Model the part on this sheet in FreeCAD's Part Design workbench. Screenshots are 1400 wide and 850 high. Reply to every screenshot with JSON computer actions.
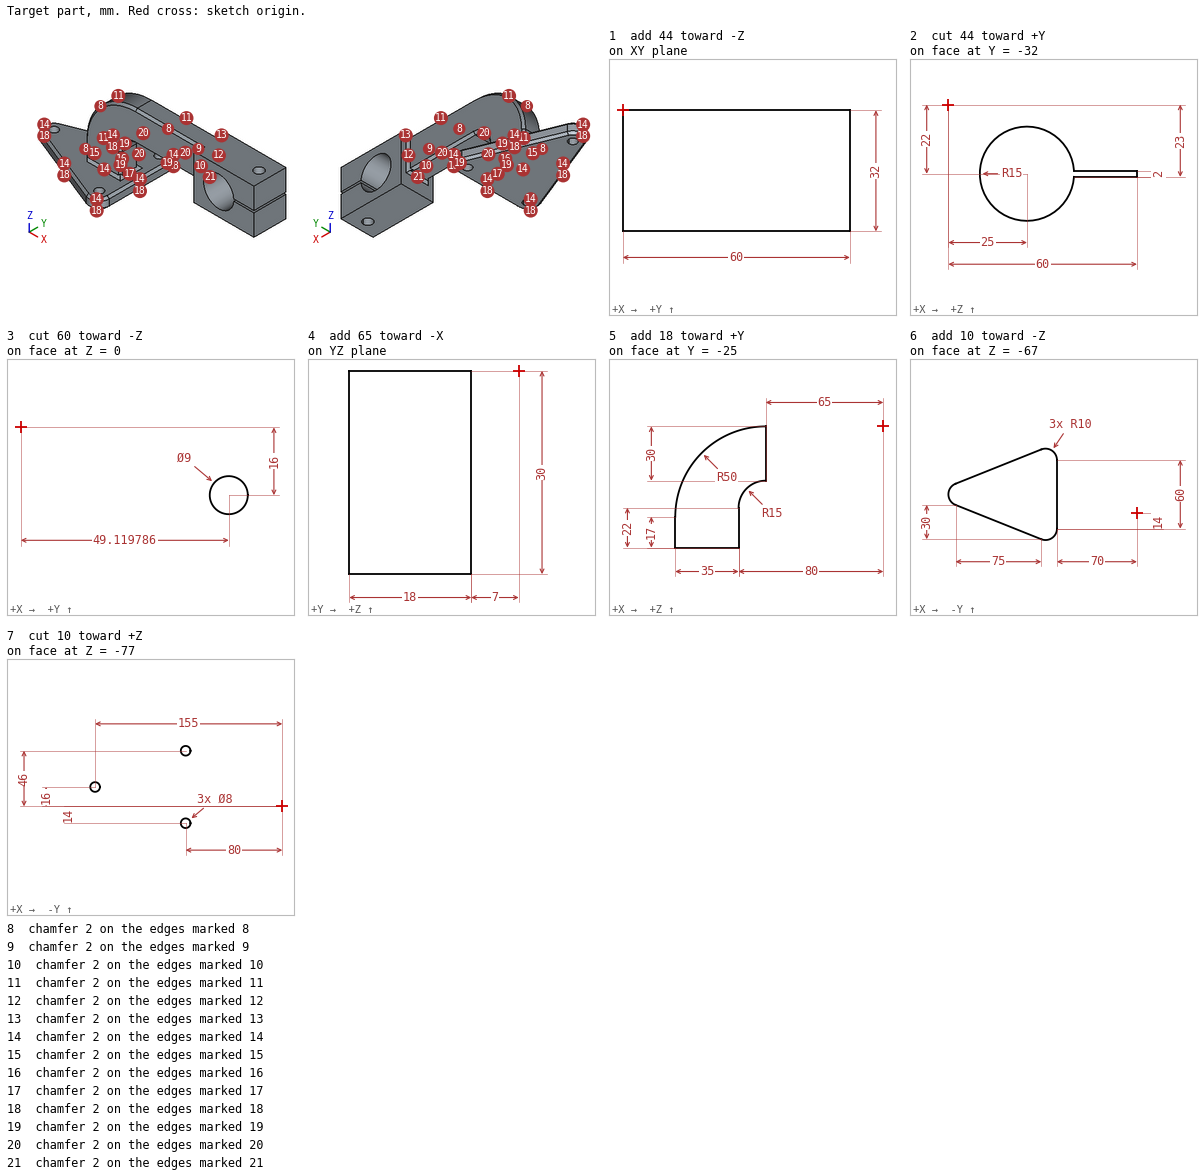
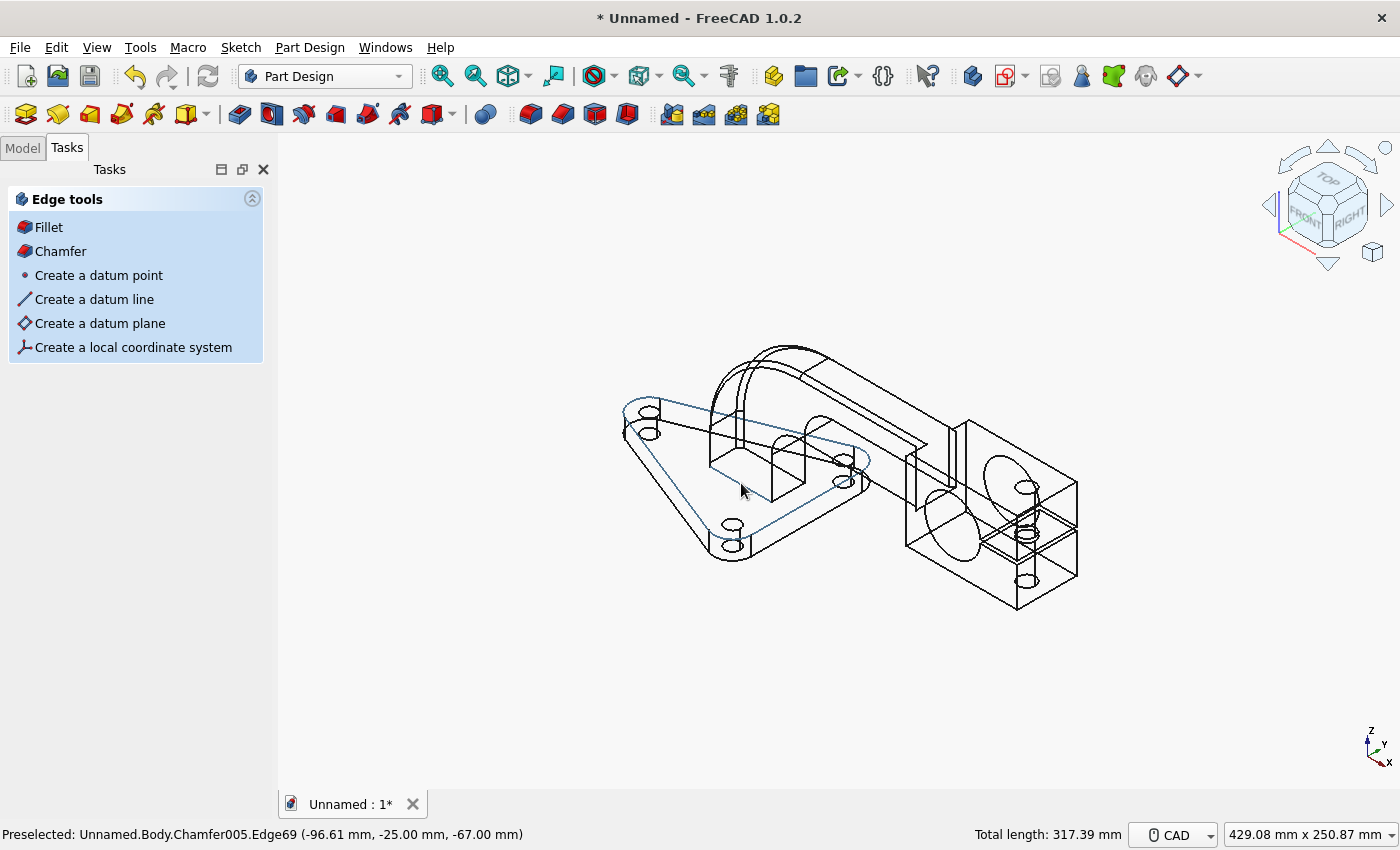
{"action": "left_click", "coordinate": [564, 114]}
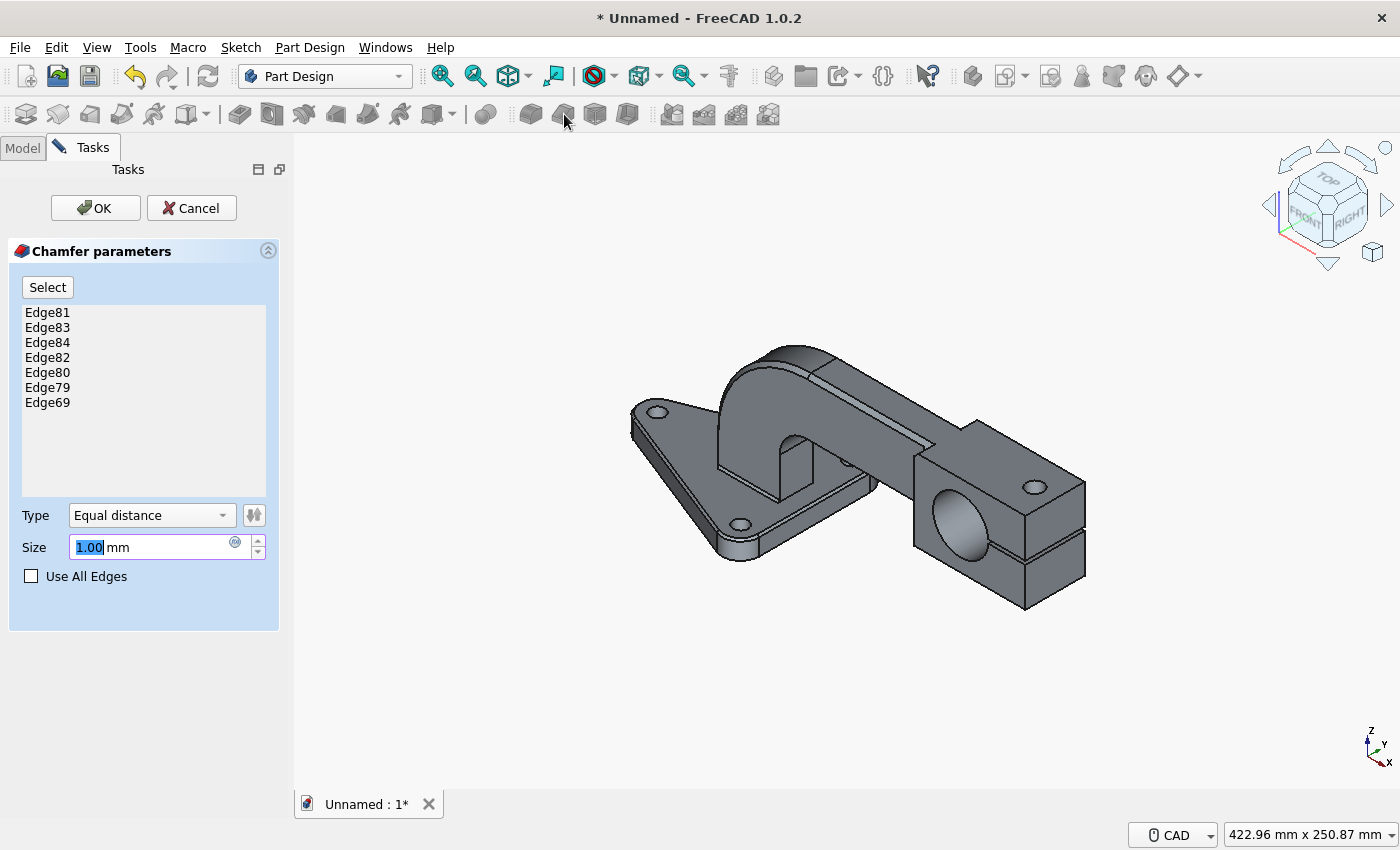
{"action": "type", "text": "2"}
{"action": "key", "text": "Tab"}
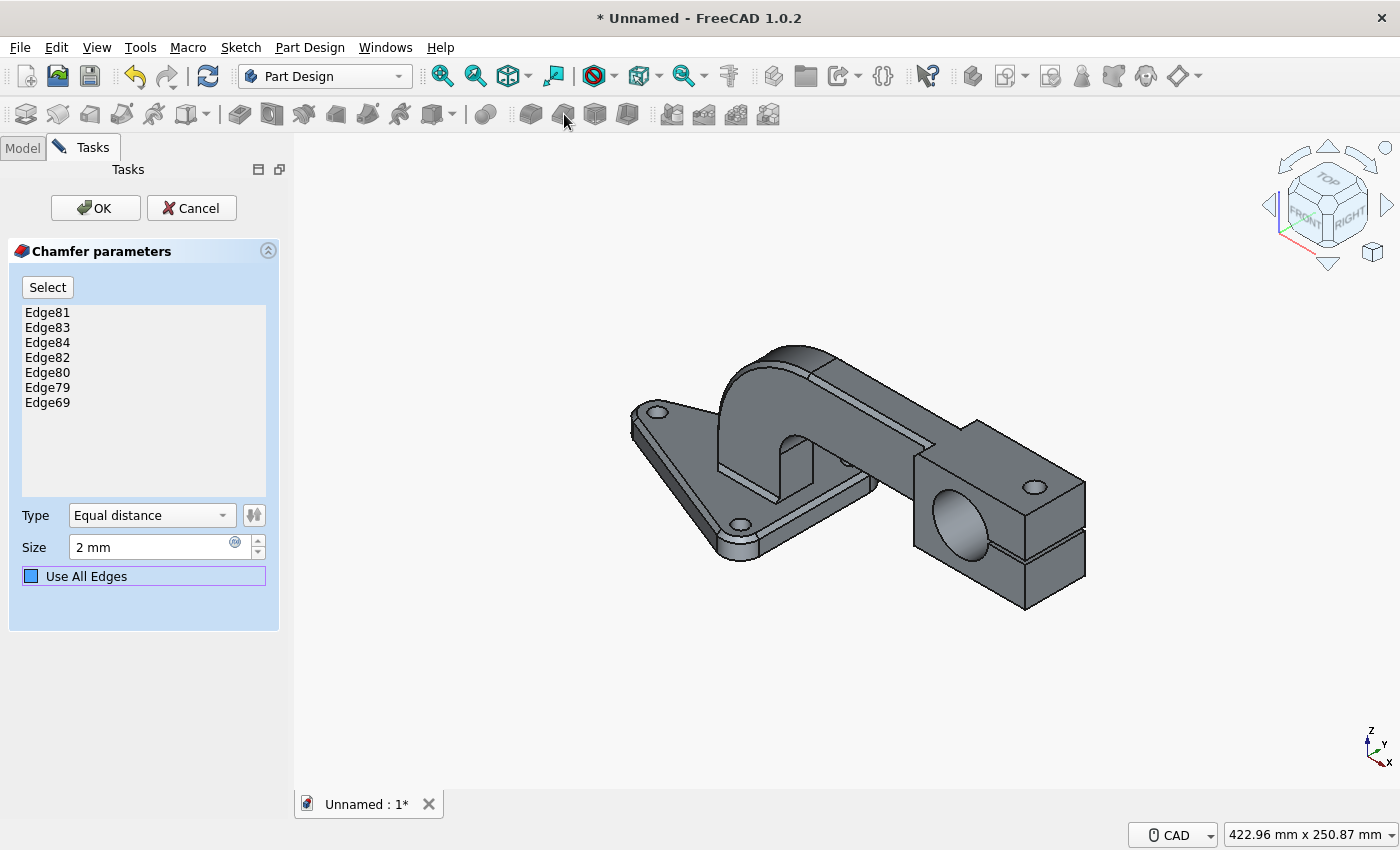
{"action": "left_click", "coordinate": [96, 208]}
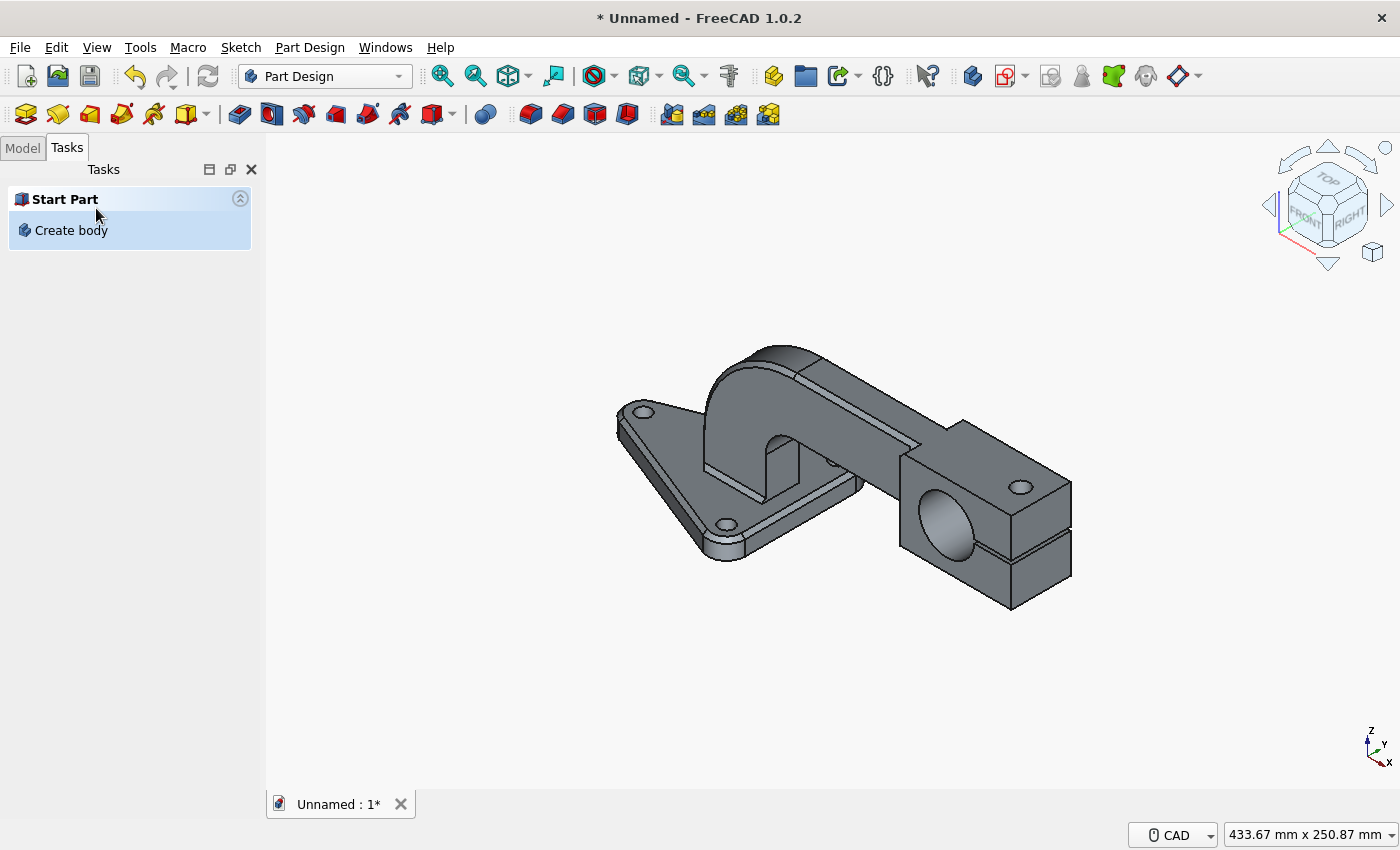
{"action": "key", "text": "2"}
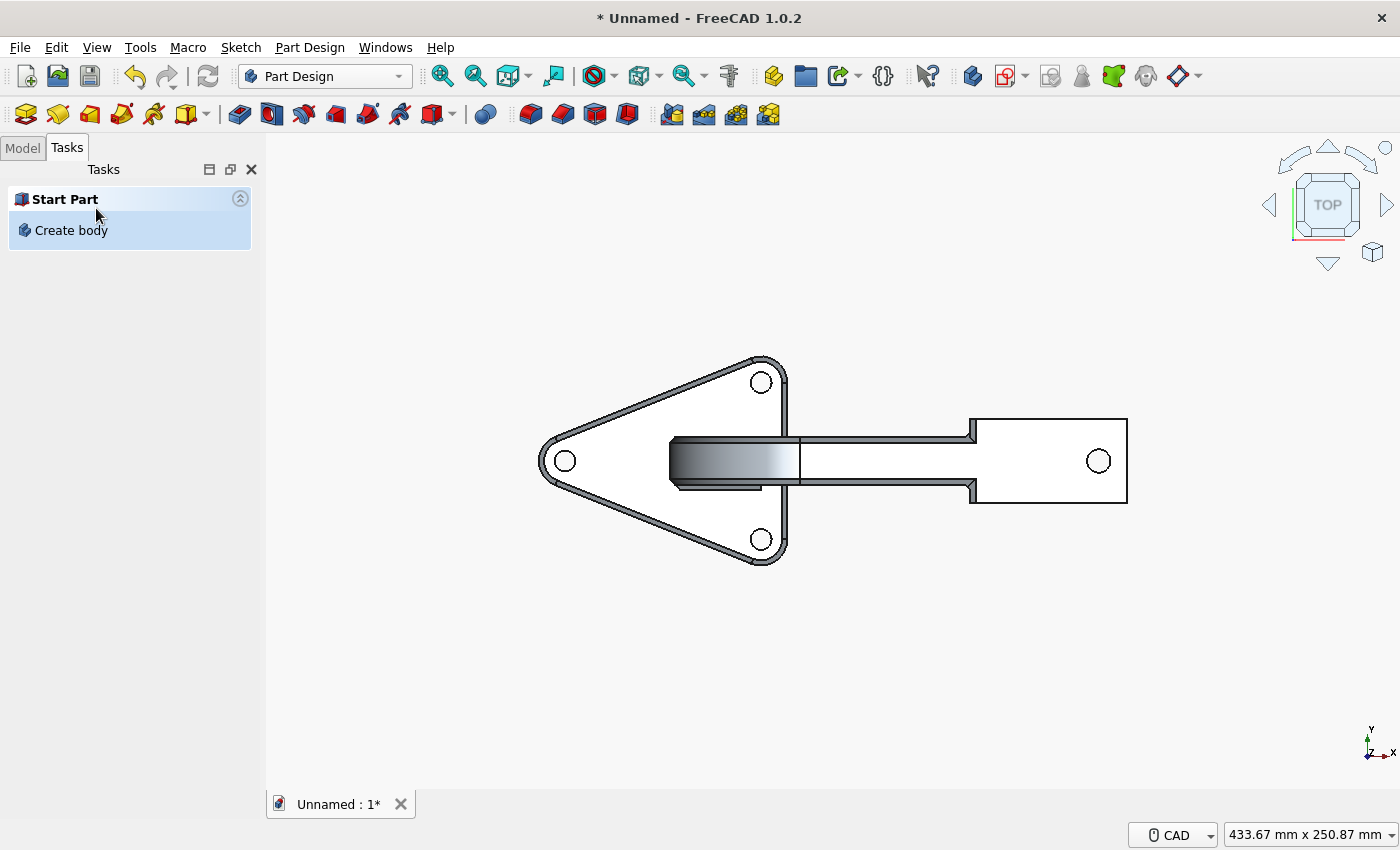
{"action": "key", "text": "0"}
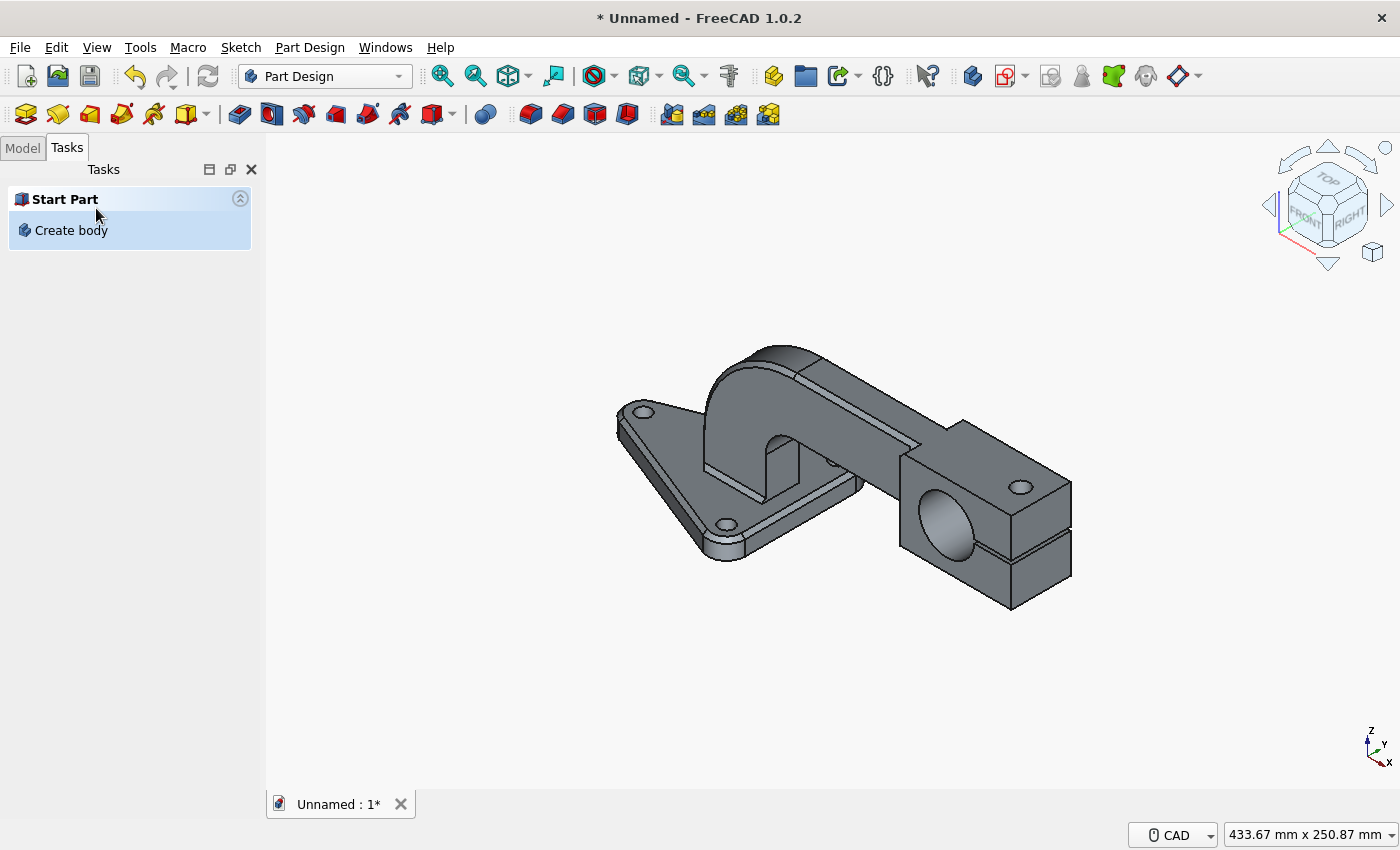
{"action": "key", "text": "1"}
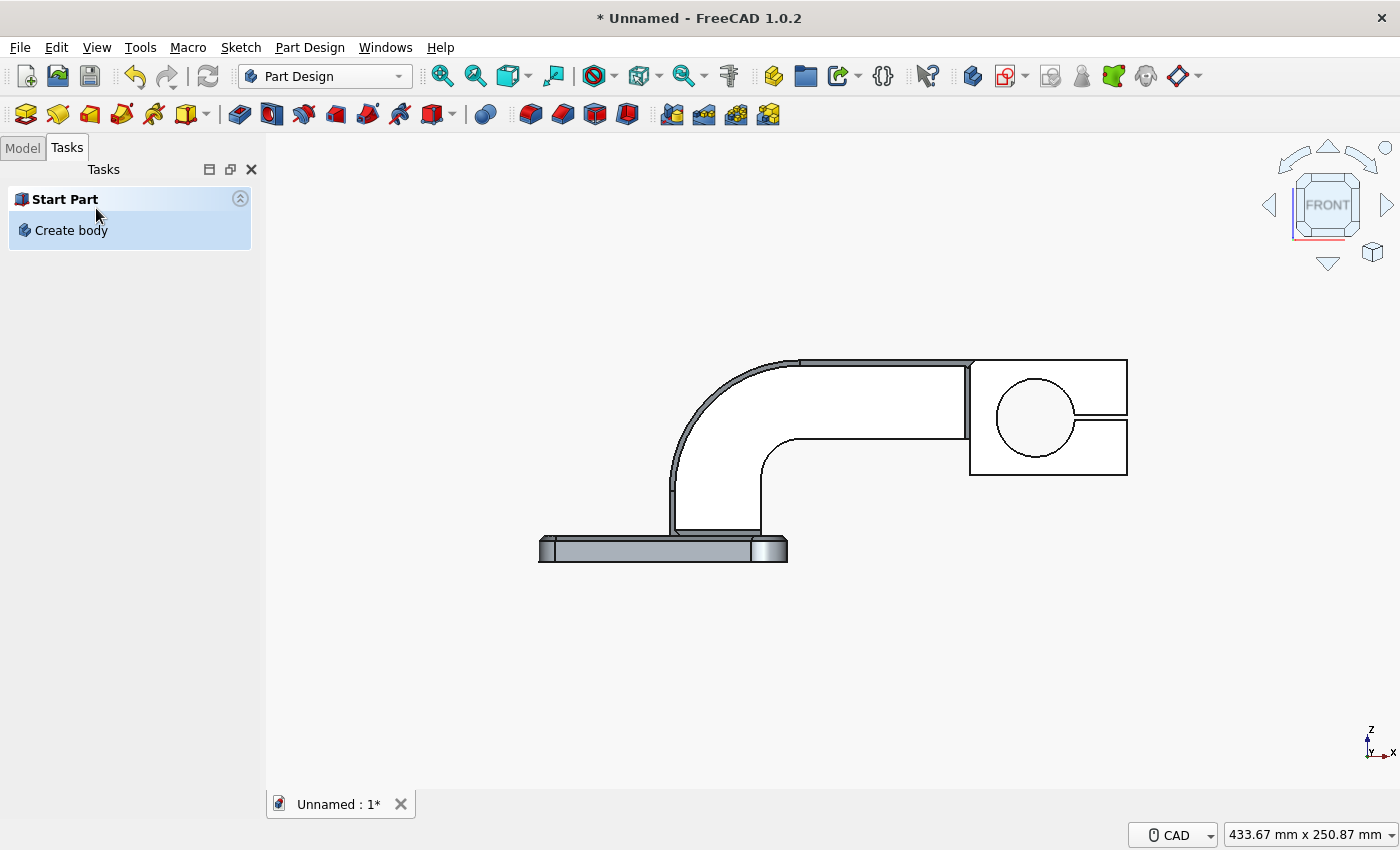
{"action": "key", "text": "3"}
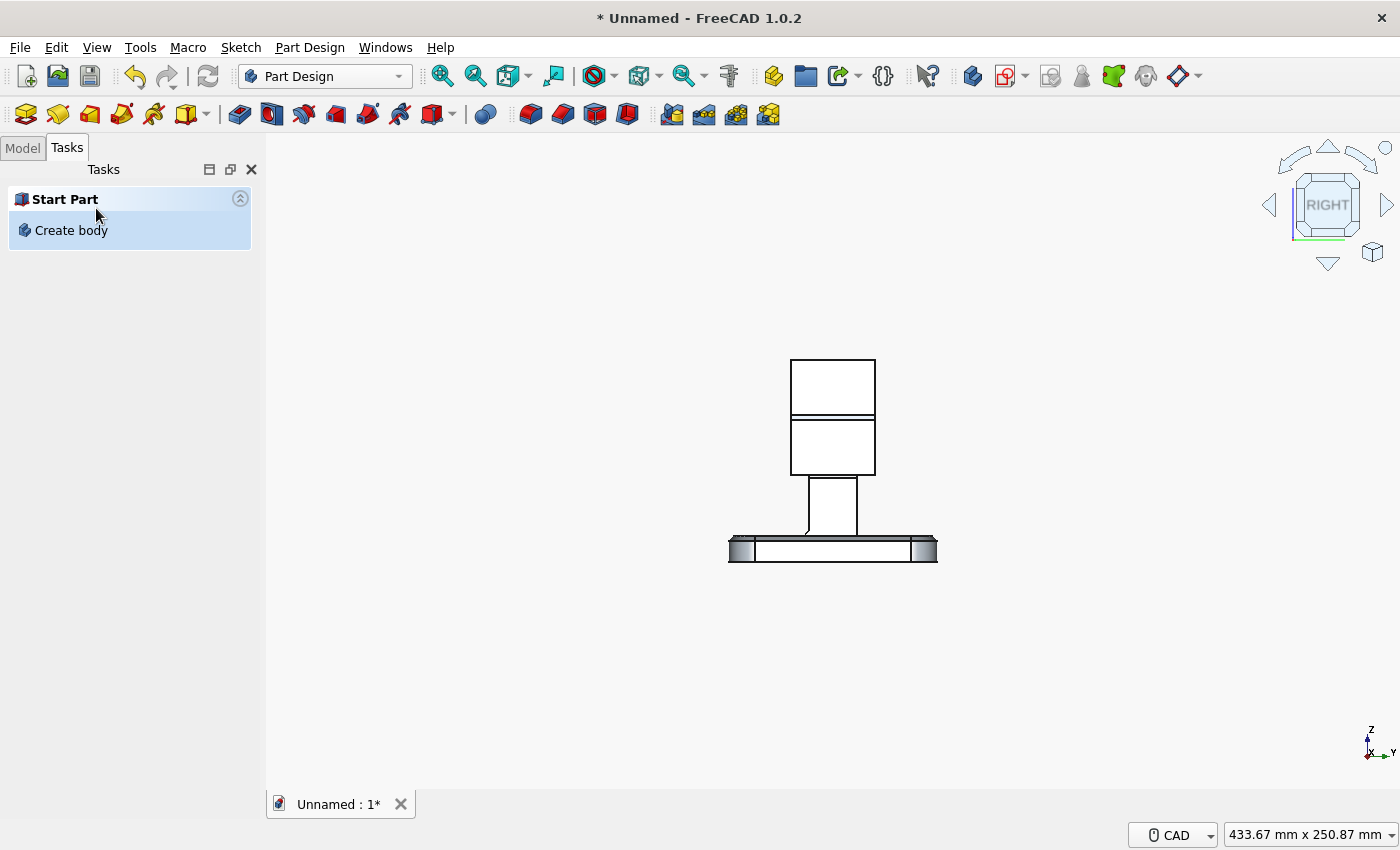
{"action": "left_click", "coordinate": [444, 76]}